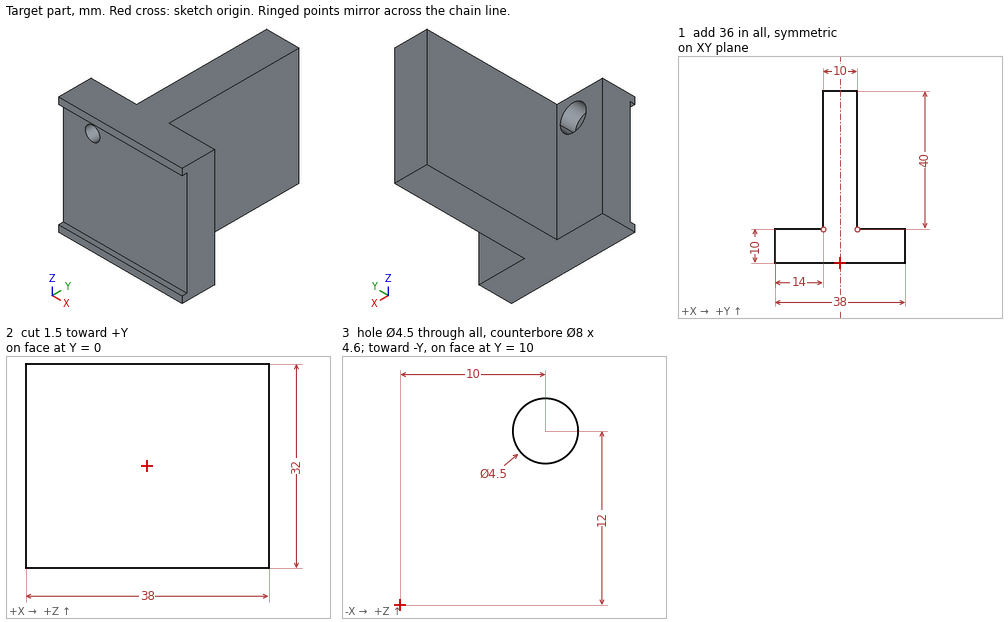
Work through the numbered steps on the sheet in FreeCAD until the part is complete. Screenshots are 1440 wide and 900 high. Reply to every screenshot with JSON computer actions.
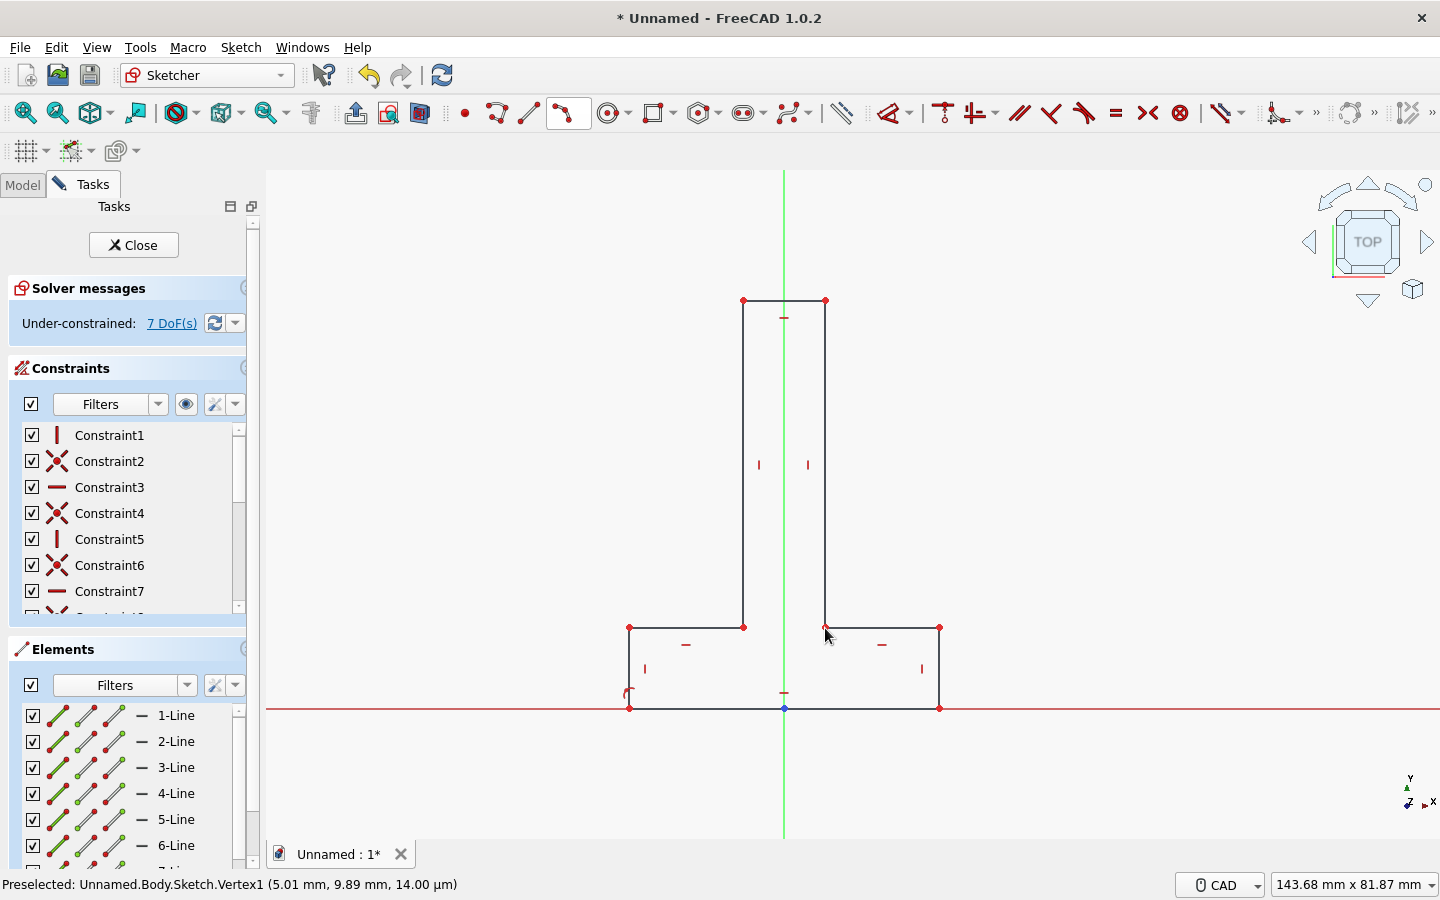
{"action": "left_click", "coordinate": [825, 628]}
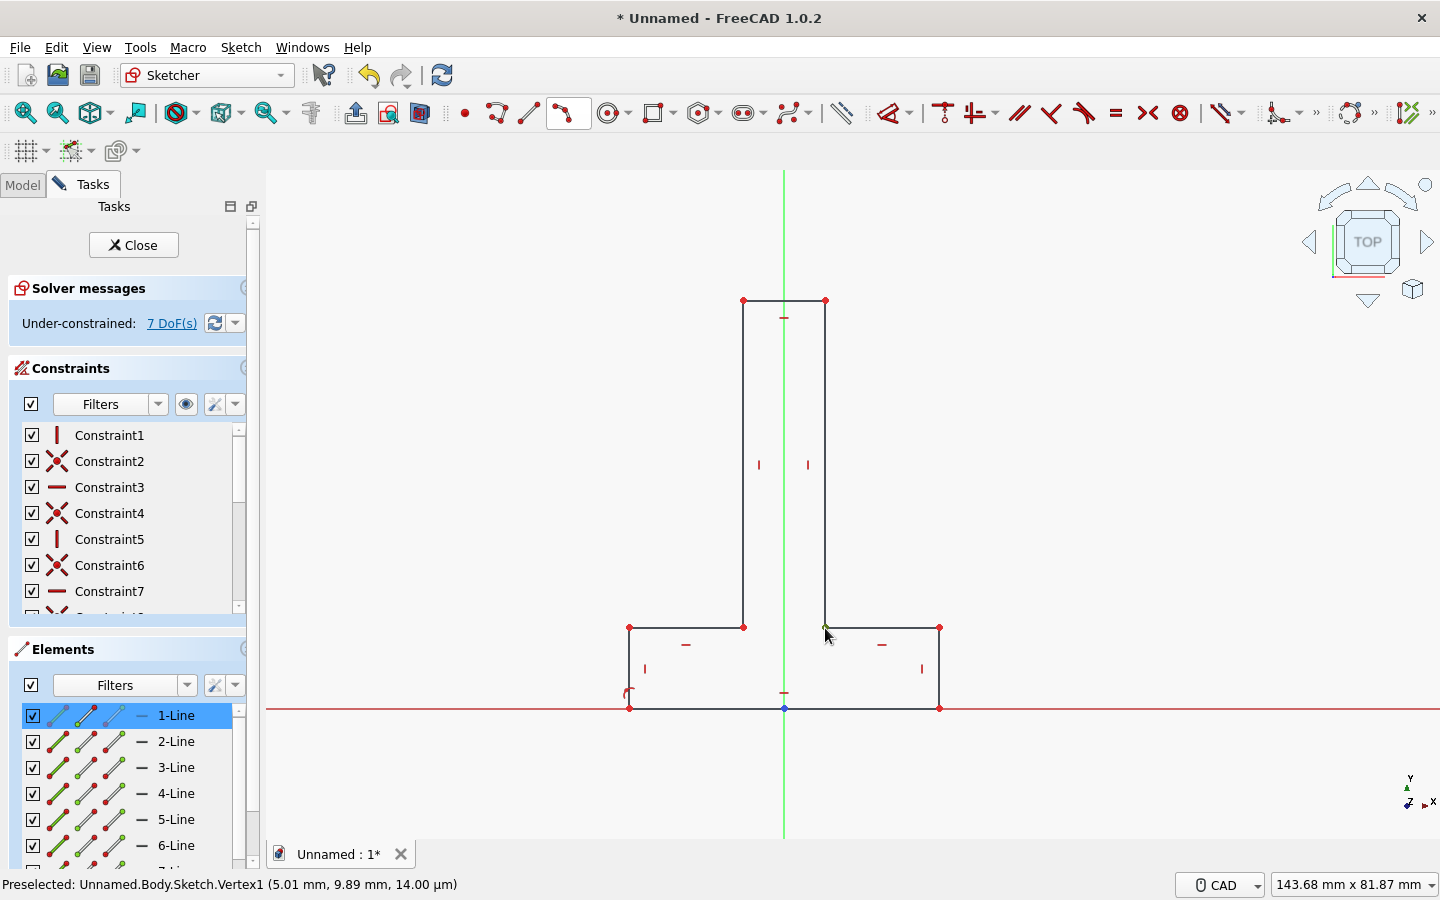
{"action": "left_click", "coordinate": [743, 628]}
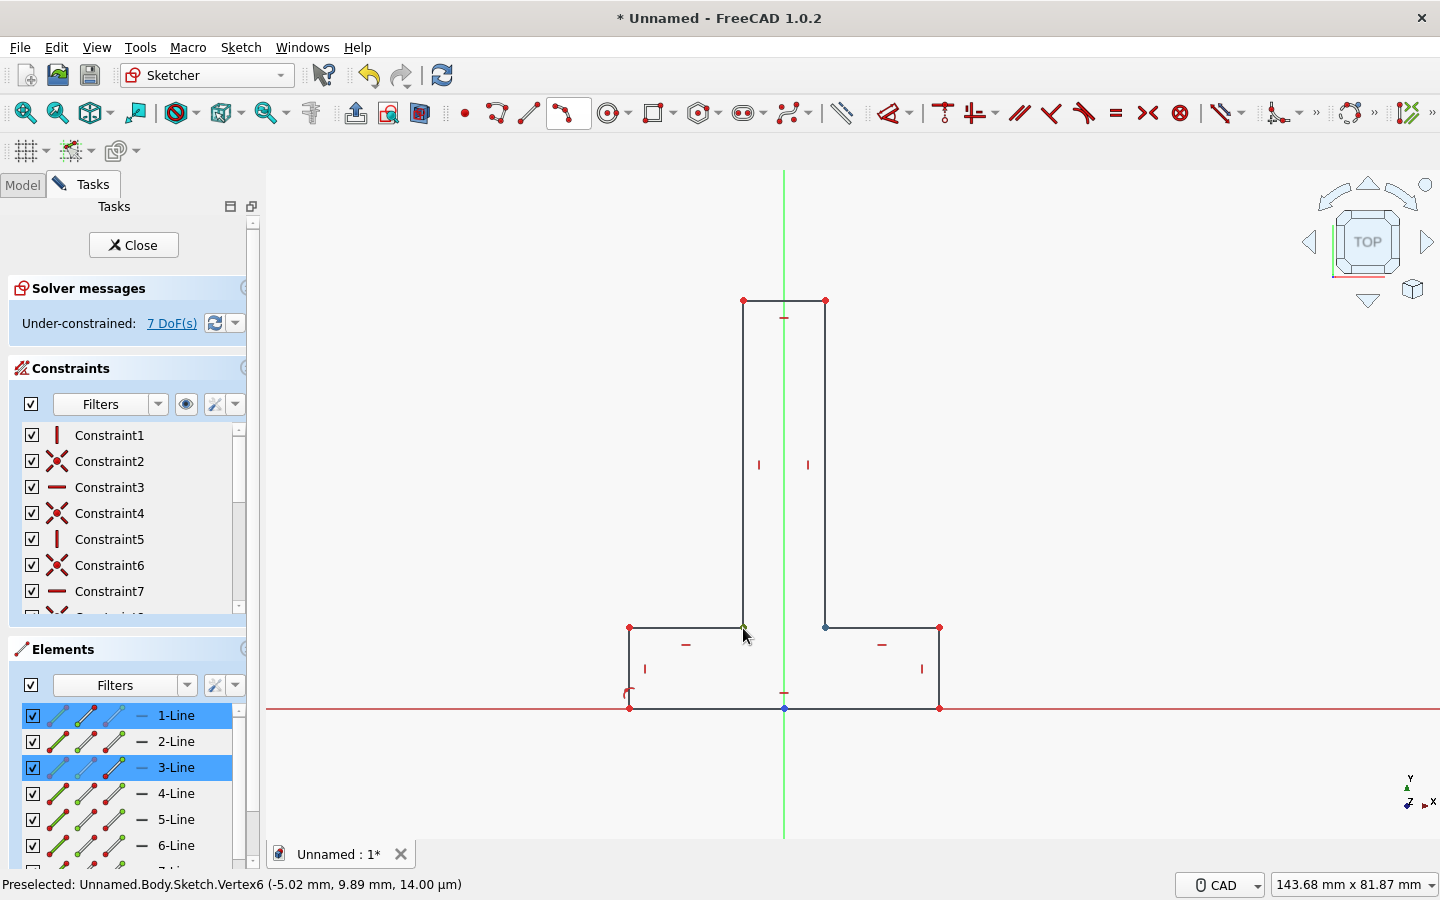
{"action": "left_click", "coordinate": [784, 767]}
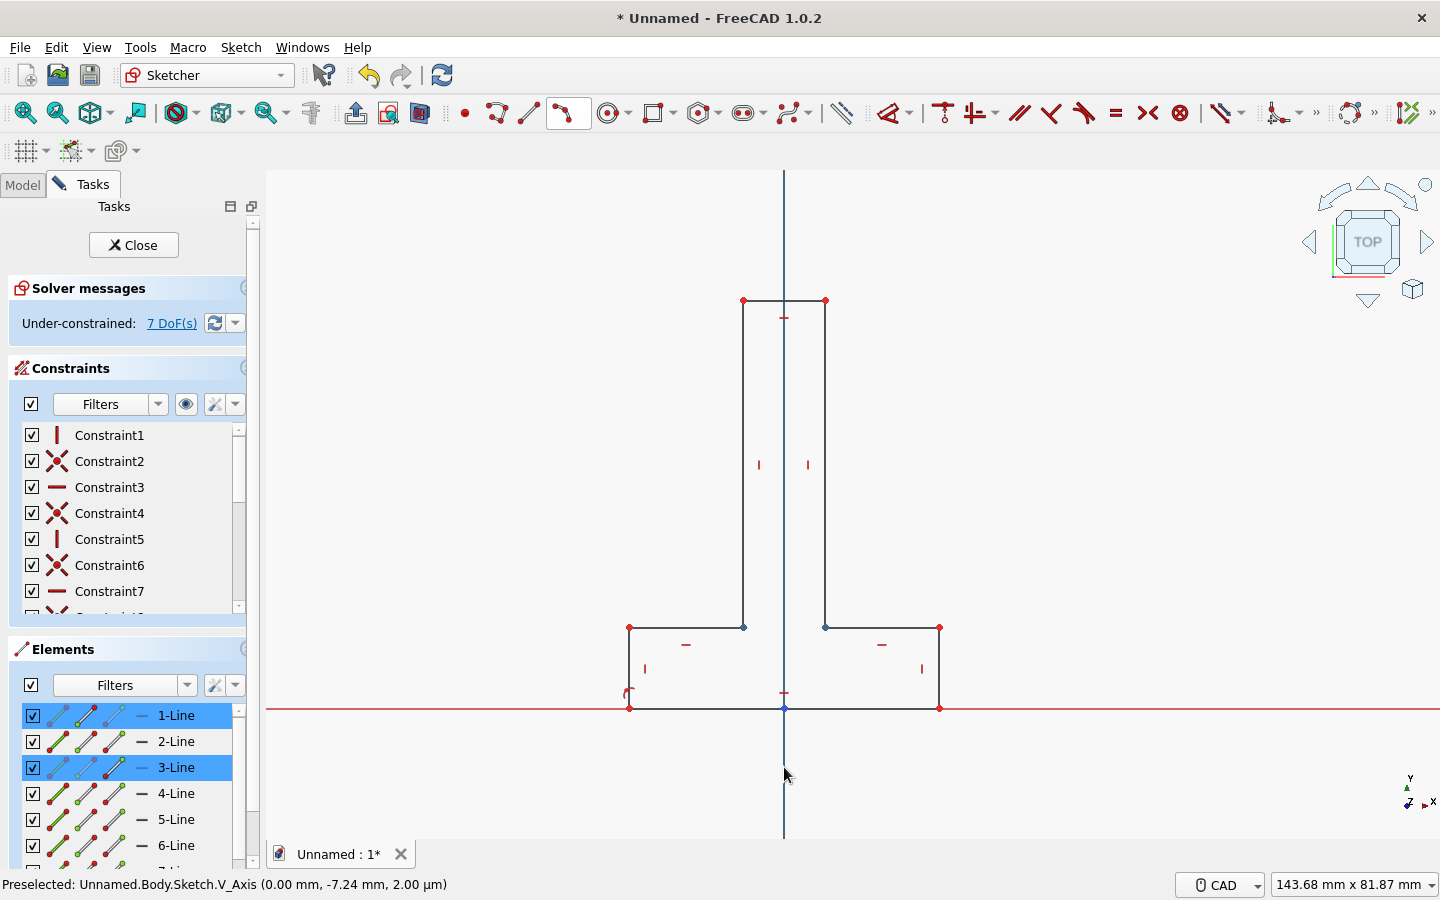
{"action": "left_click", "coordinate": [1148, 114]}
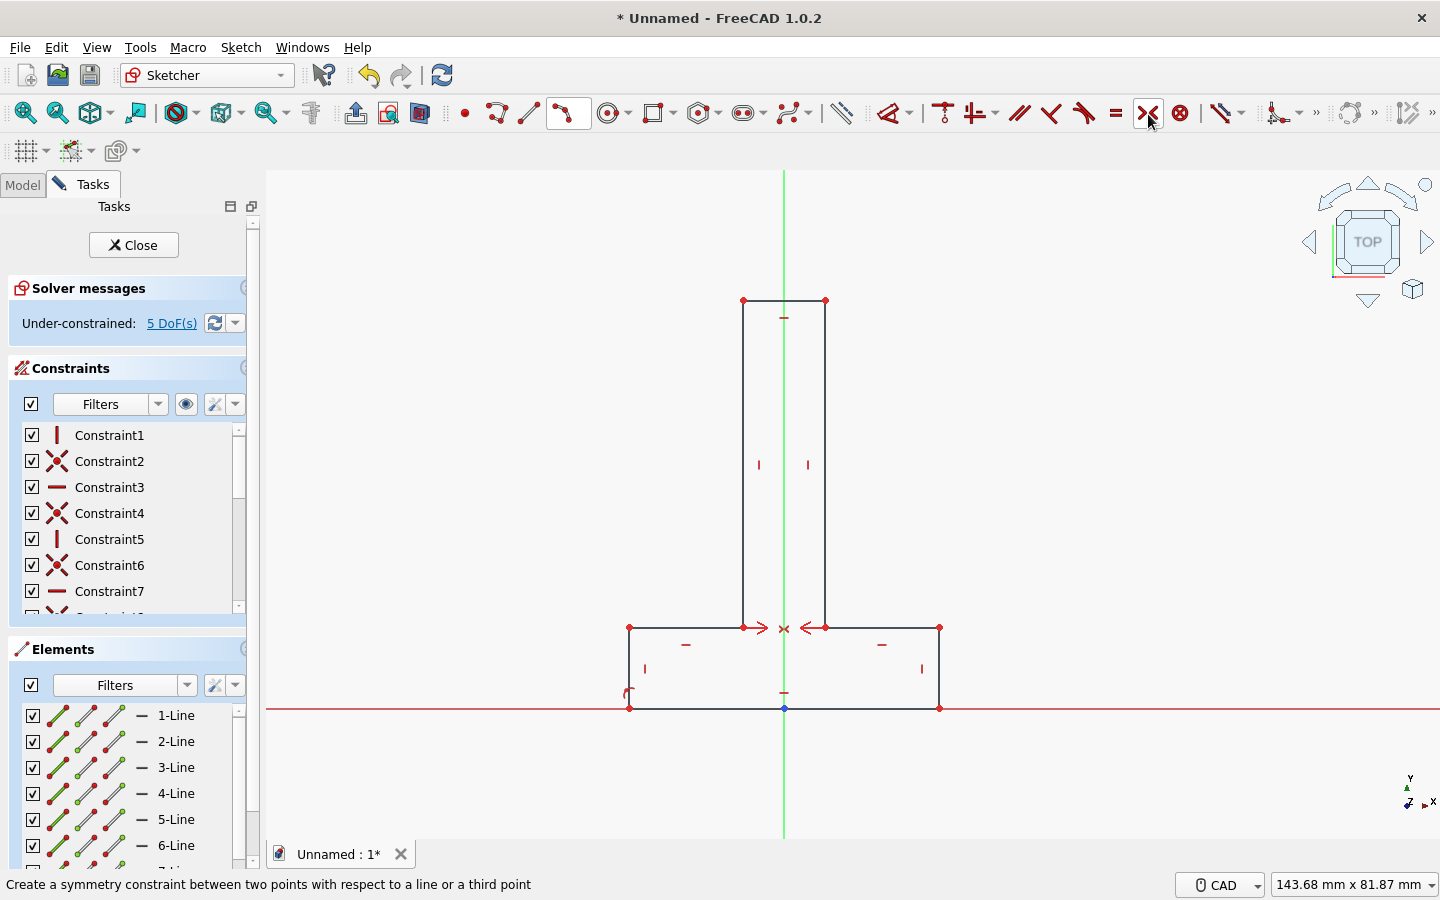
{"action": "left_click", "coordinate": [888, 114]}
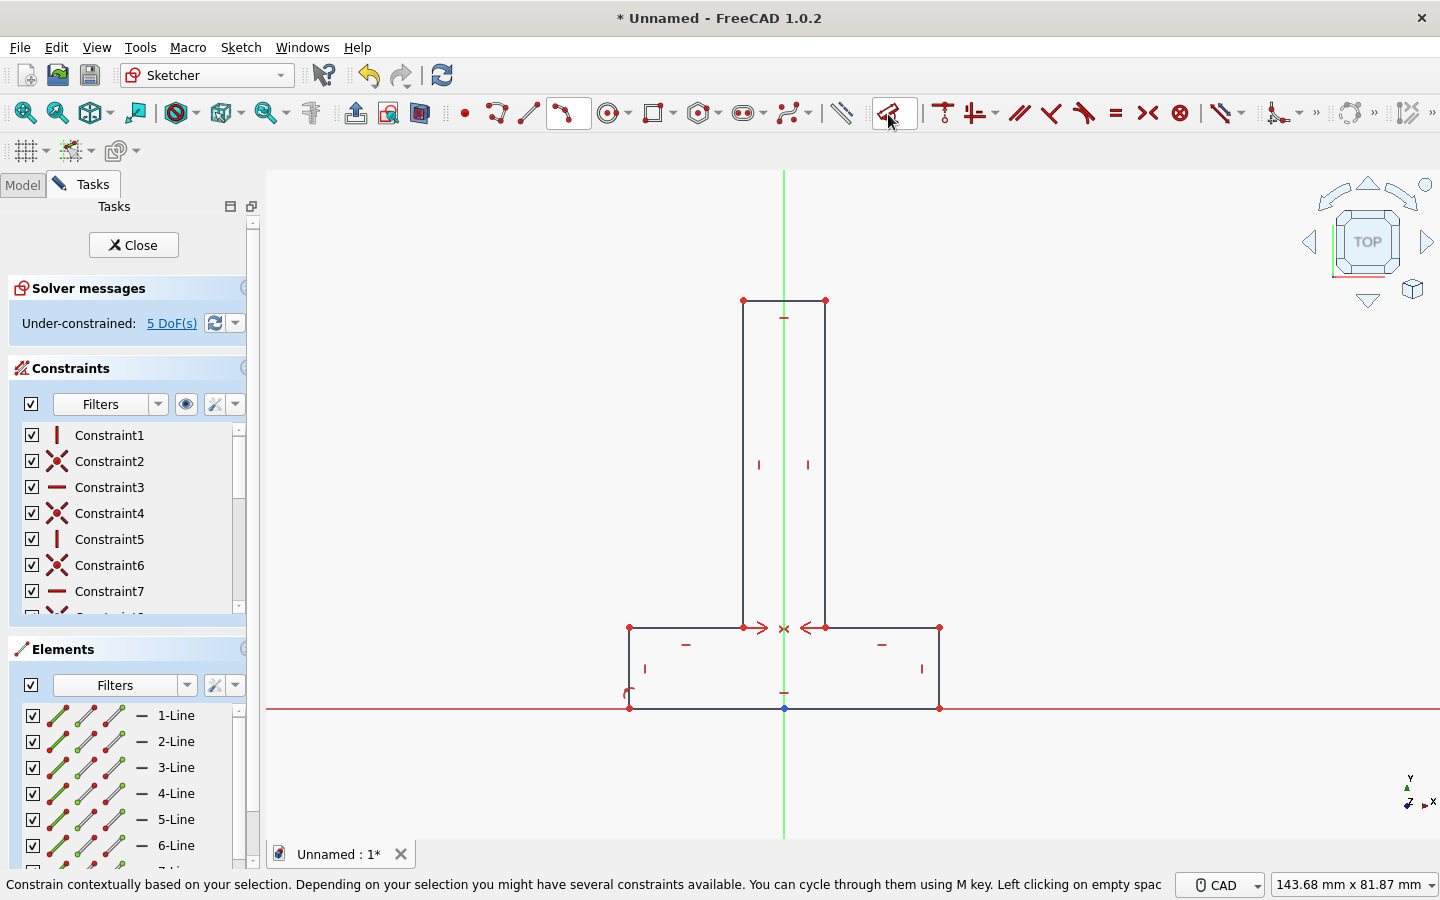
{"action": "left_click", "coordinate": [825, 530]}
{"action": "left_click", "coordinate": [859, 465]}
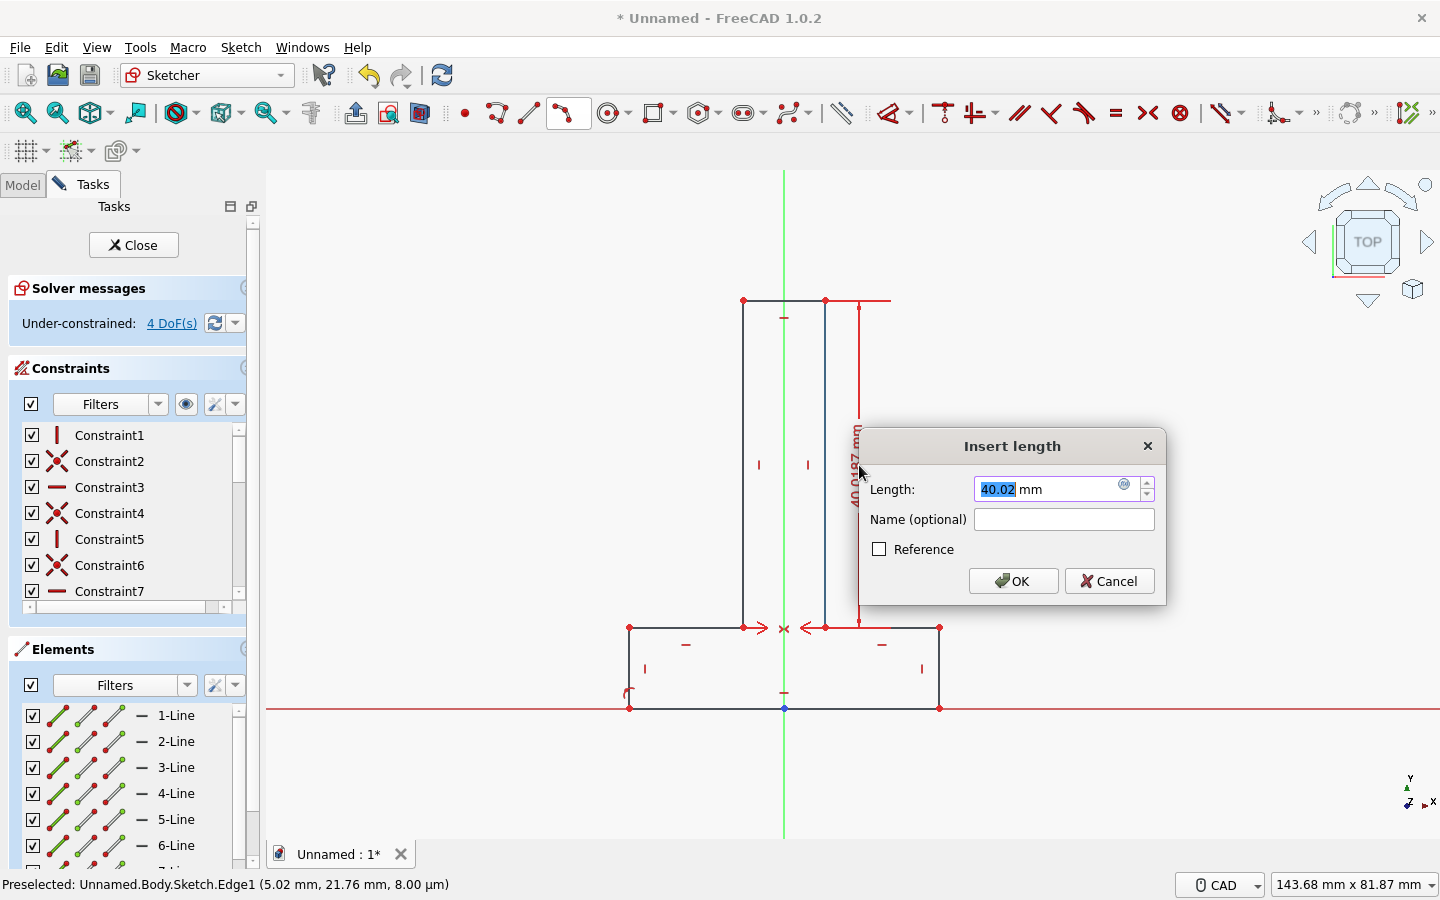
{"action": "type", "text": "40"}
{"action": "key", "text": "Return"}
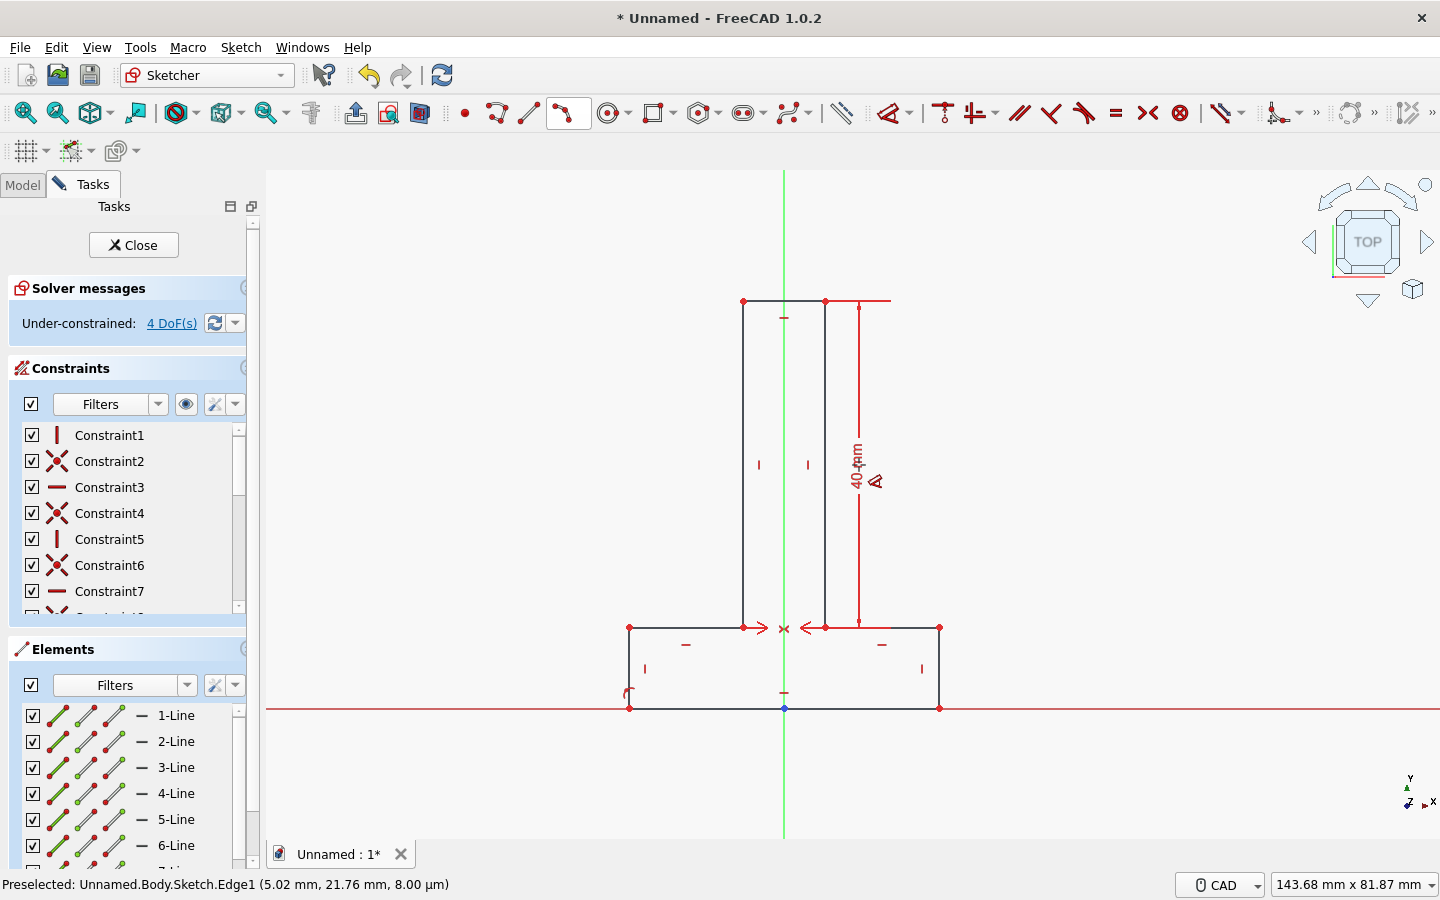
{"action": "left_click", "coordinate": [800, 301]}
{"action": "left_click", "coordinate": [765, 267]}